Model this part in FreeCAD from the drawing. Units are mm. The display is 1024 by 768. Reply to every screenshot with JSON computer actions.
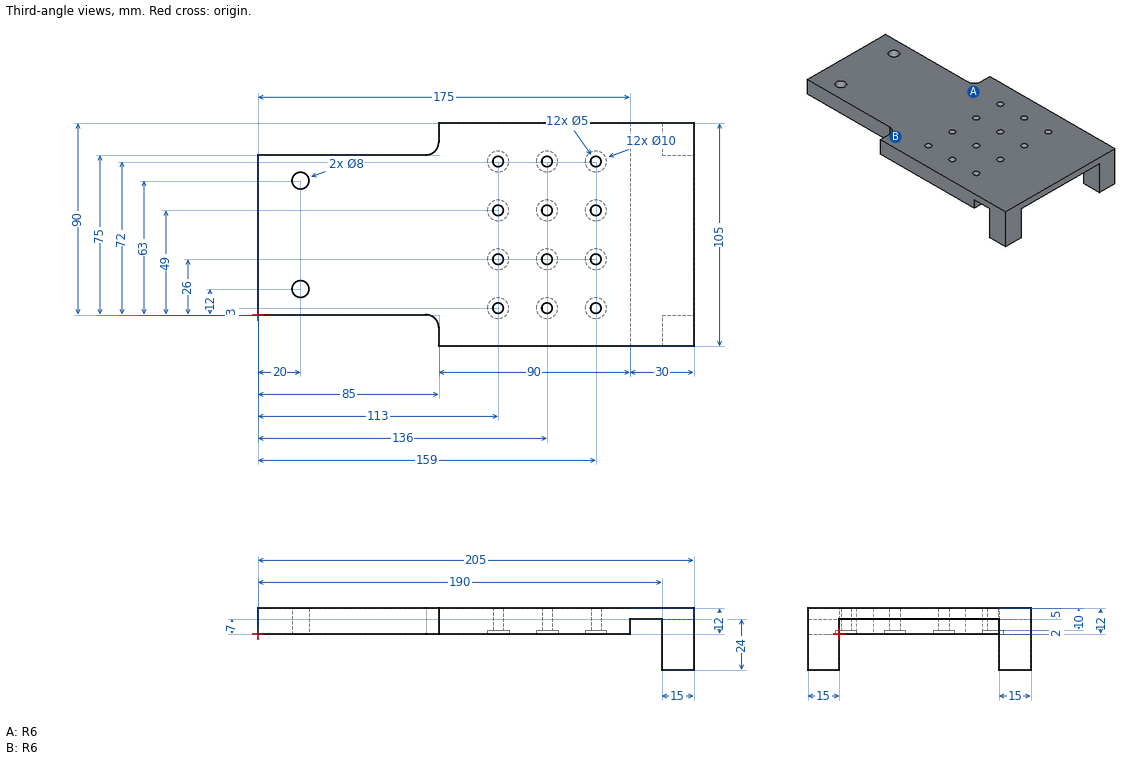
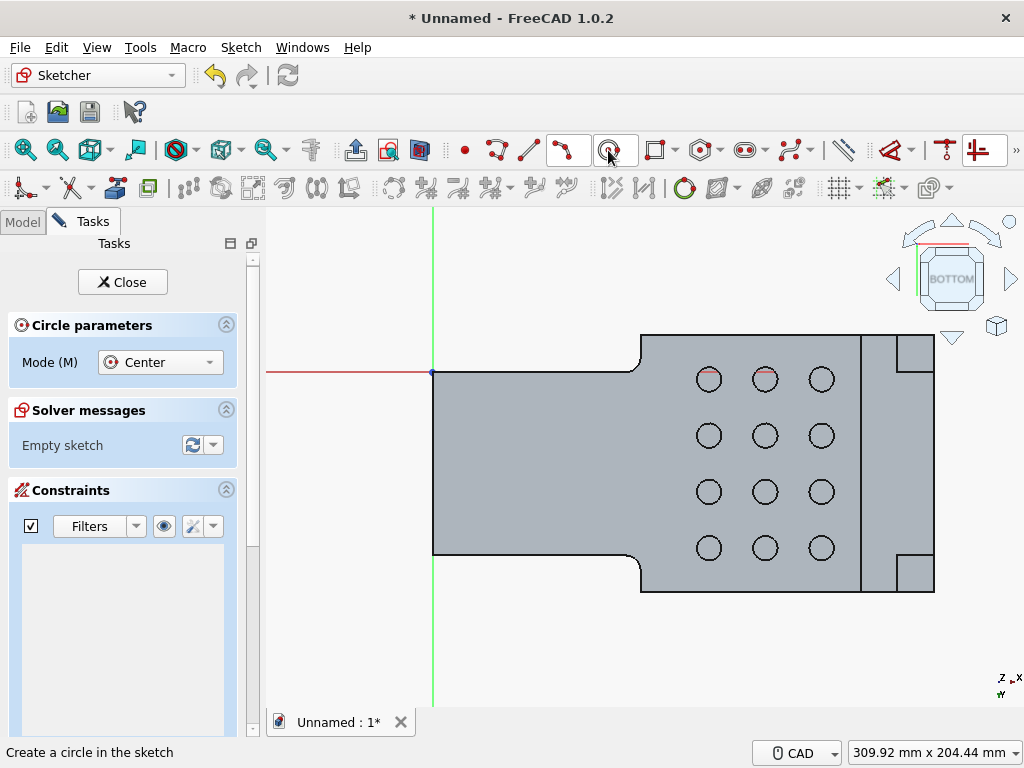
{"action": "scroll", "coordinate": [822, 548], "scroll_direction": "up", "scroll_amount": 7}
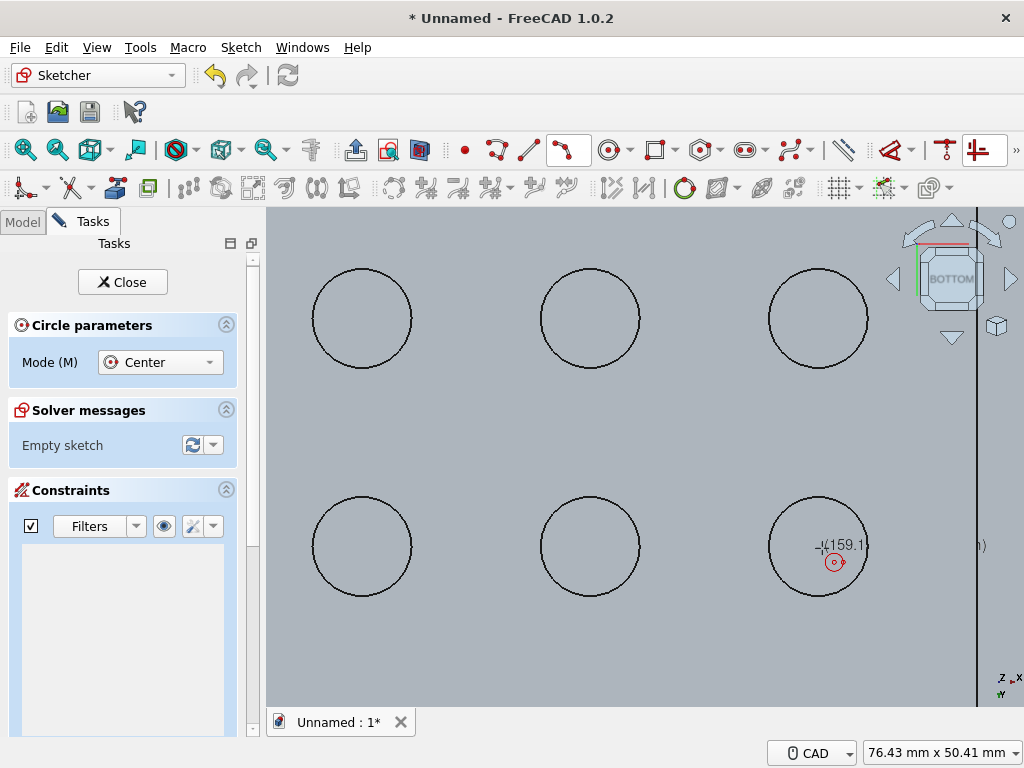
{"action": "scroll", "coordinate": [751, 540], "scroll_direction": "down", "scroll_amount": 7}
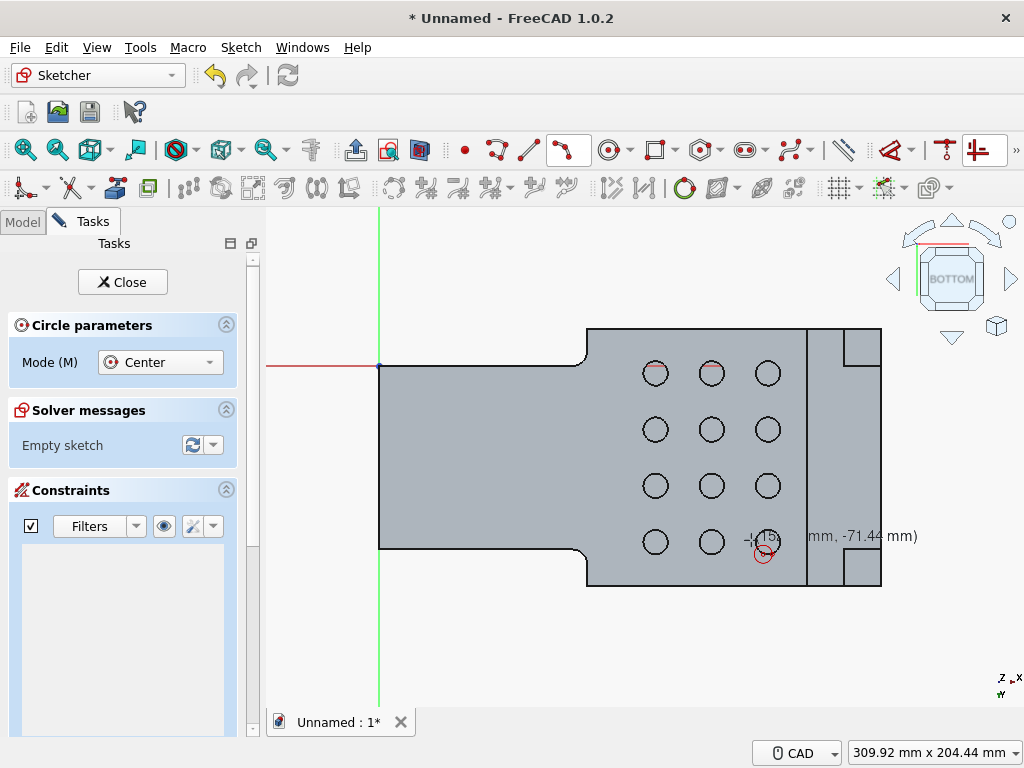
{"action": "left_click", "coordinate": [768, 542]}
{"action": "mouse_move", "coordinate": [772, 538]}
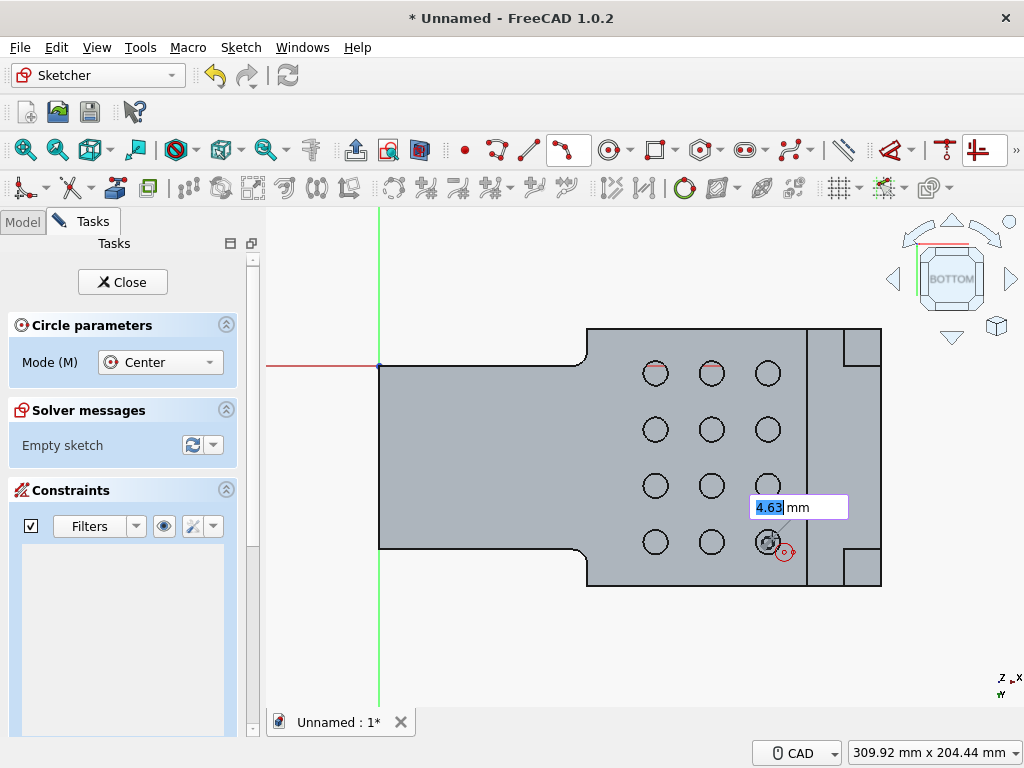
{"action": "type", "text": "5"}
{"action": "key", "text": "Return"}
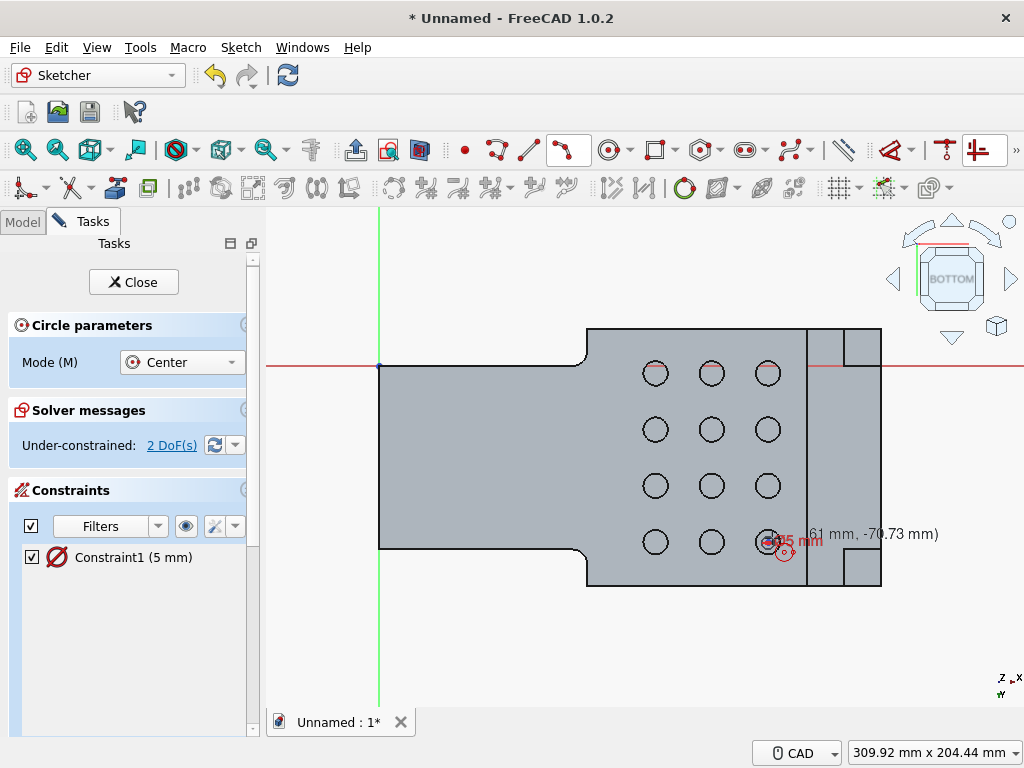
{"action": "scroll", "coordinate": [712, 542], "scroll_direction": "up", "scroll_amount": 7}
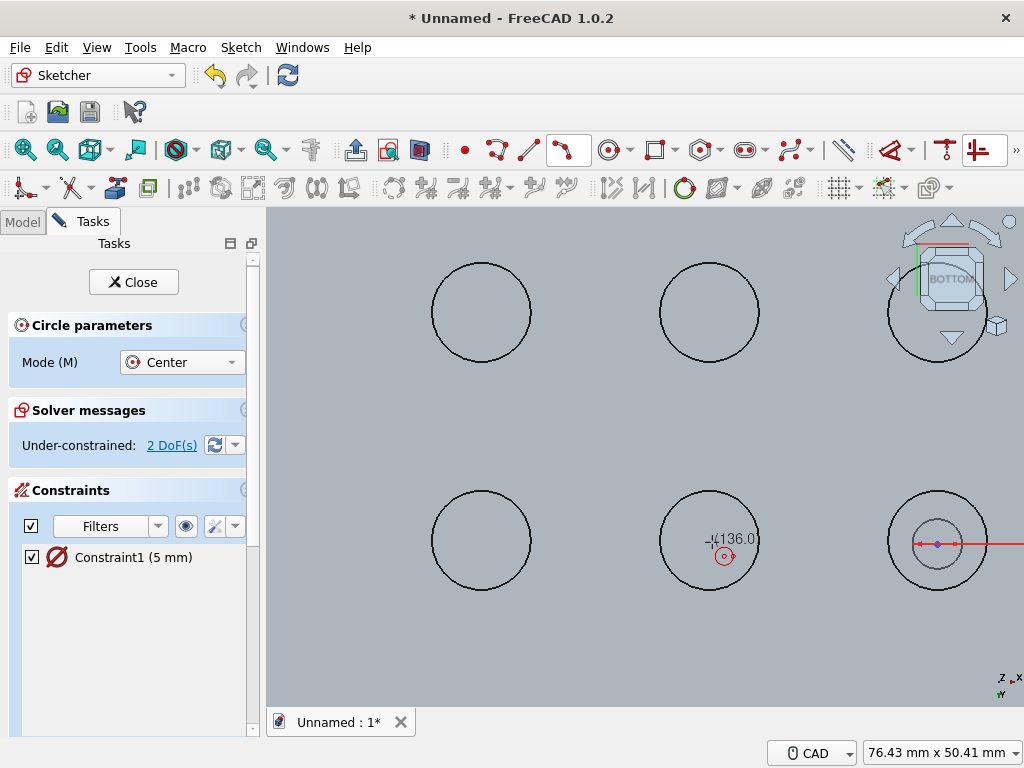
{"action": "scroll", "coordinate": [712, 543], "scroll_direction": "down", "scroll_amount": 7}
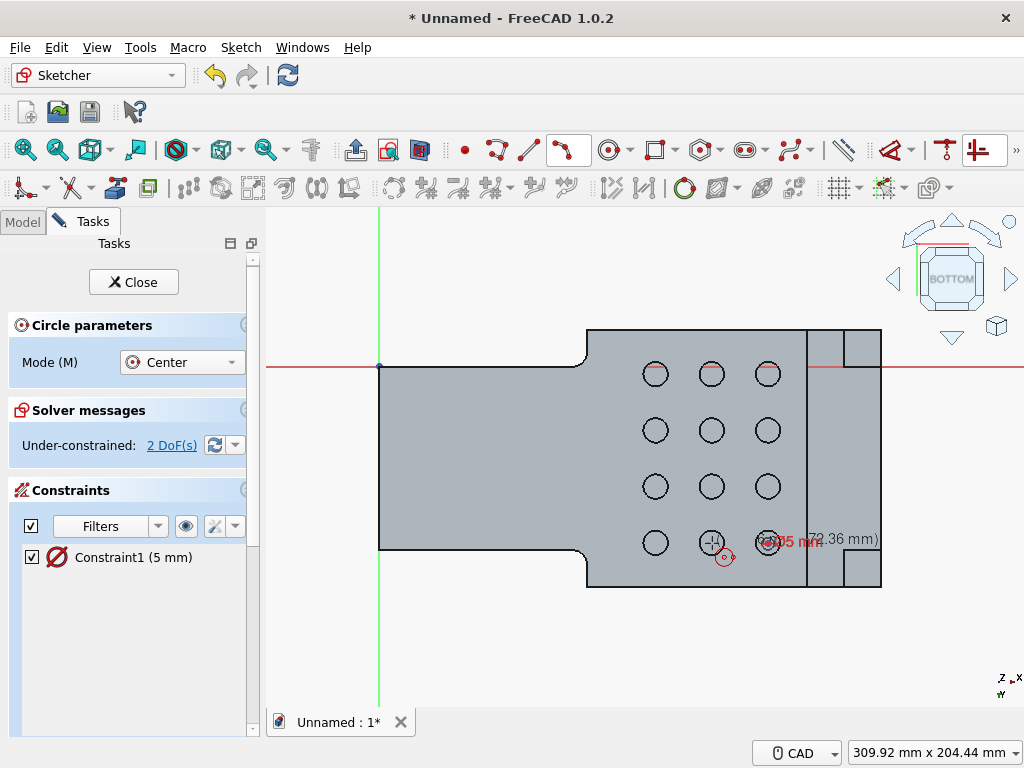
{"action": "left_click", "coordinate": [712, 543]}
{"action": "mouse_move", "coordinate": [716, 539]}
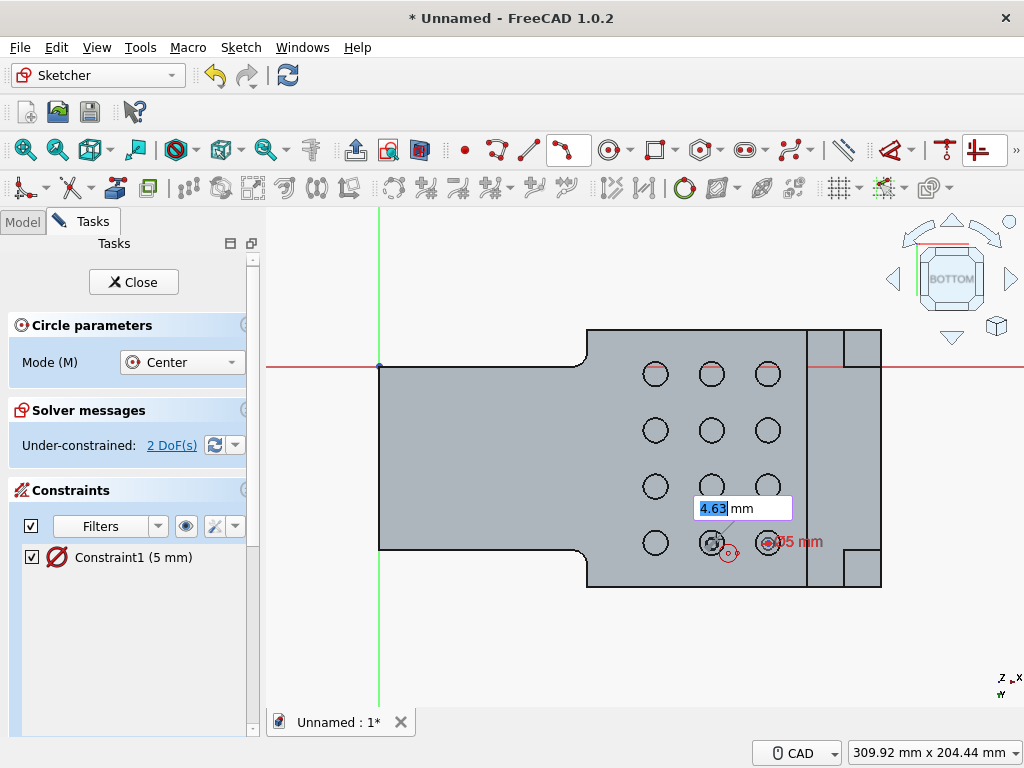
{"action": "type", "text": "5"}
{"action": "key", "text": "Return"}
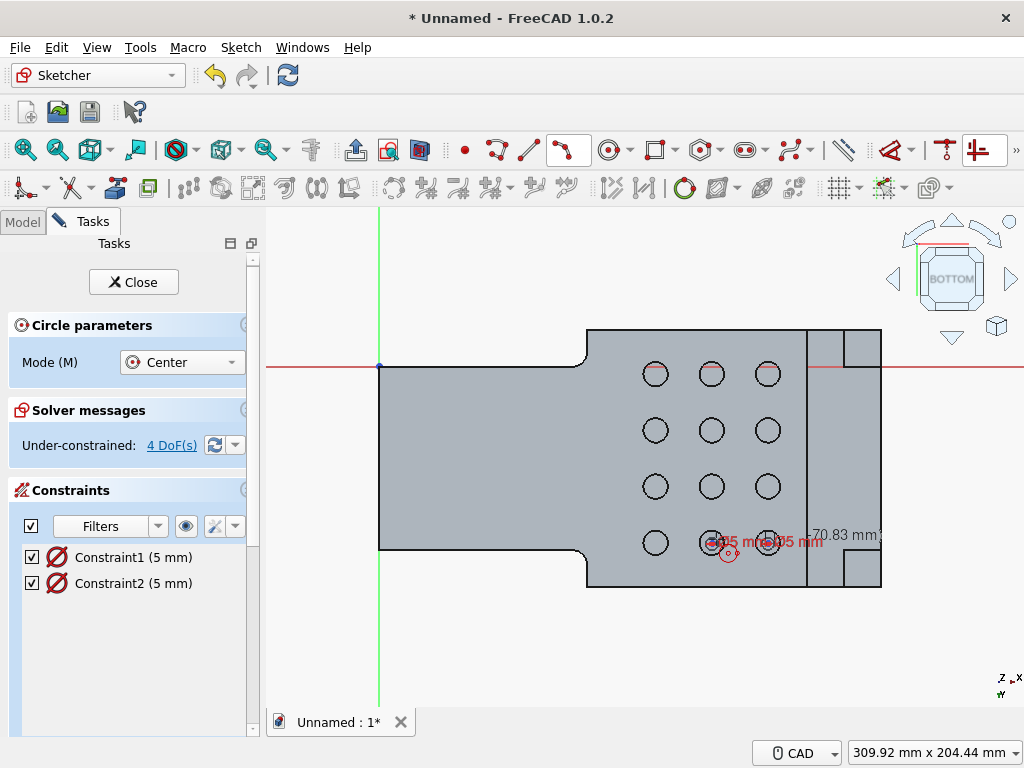
{"action": "scroll", "coordinate": [656, 543], "scroll_direction": "up", "scroll_amount": 7}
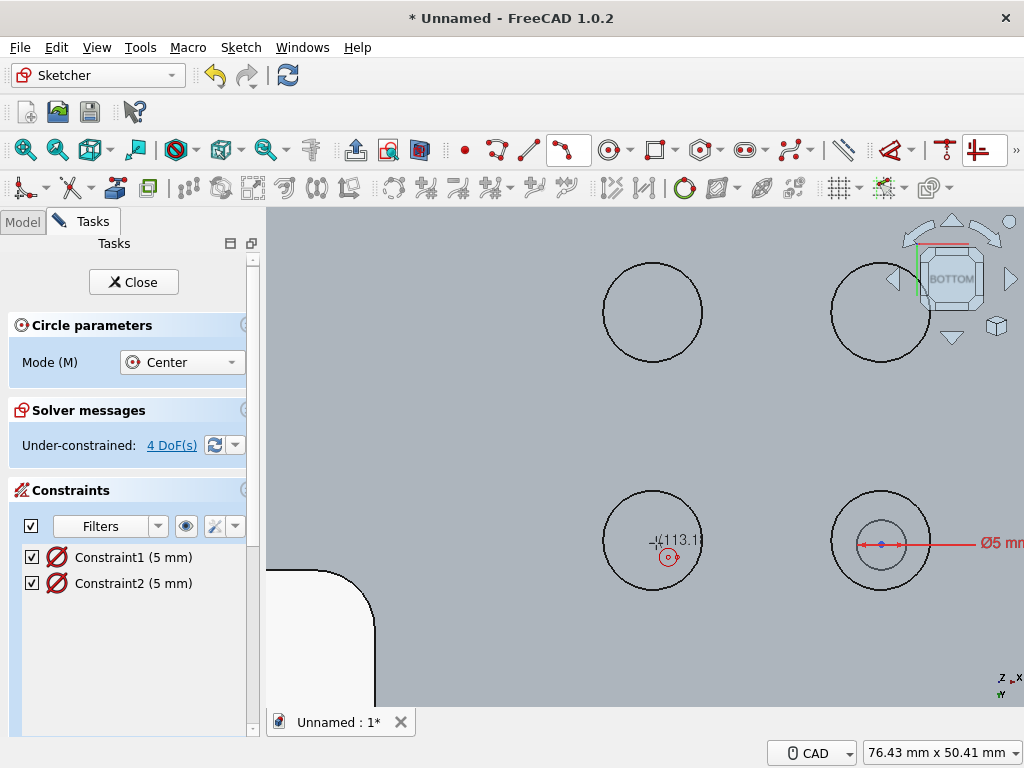
{"action": "scroll", "coordinate": [656, 543], "scroll_direction": "down", "scroll_amount": 7}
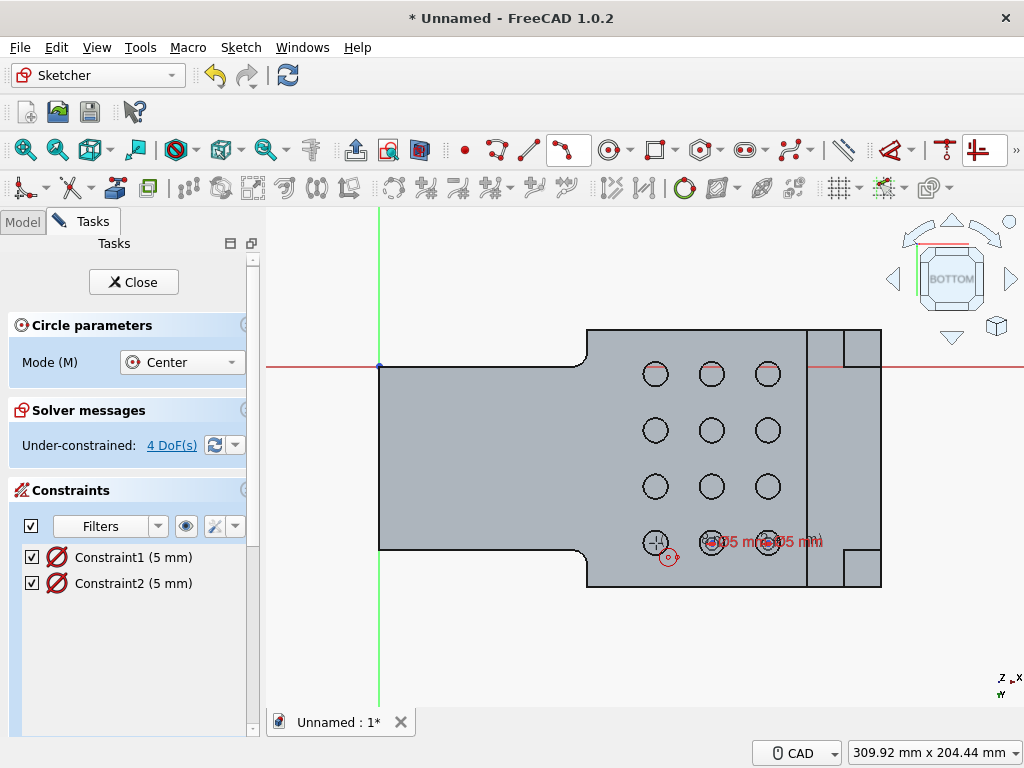
{"action": "left_click", "coordinate": [656, 543]}
{"action": "mouse_move", "coordinate": [660, 539]}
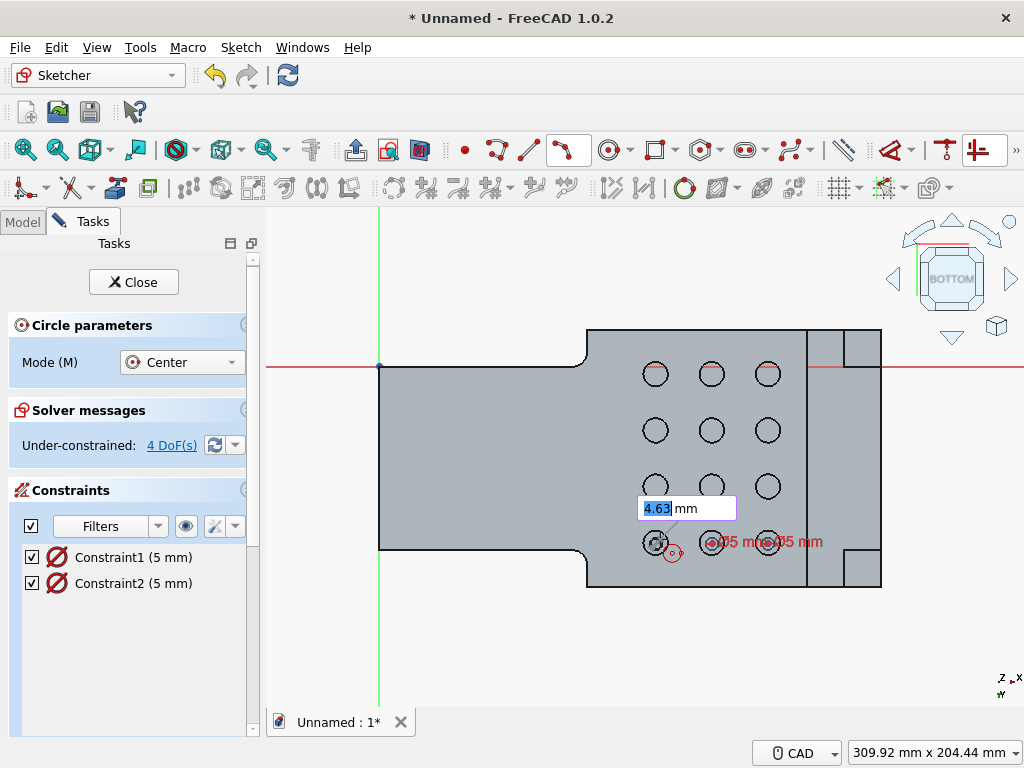
{"action": "type", "text": "5"}
{"action": "key", "text": "Return"}